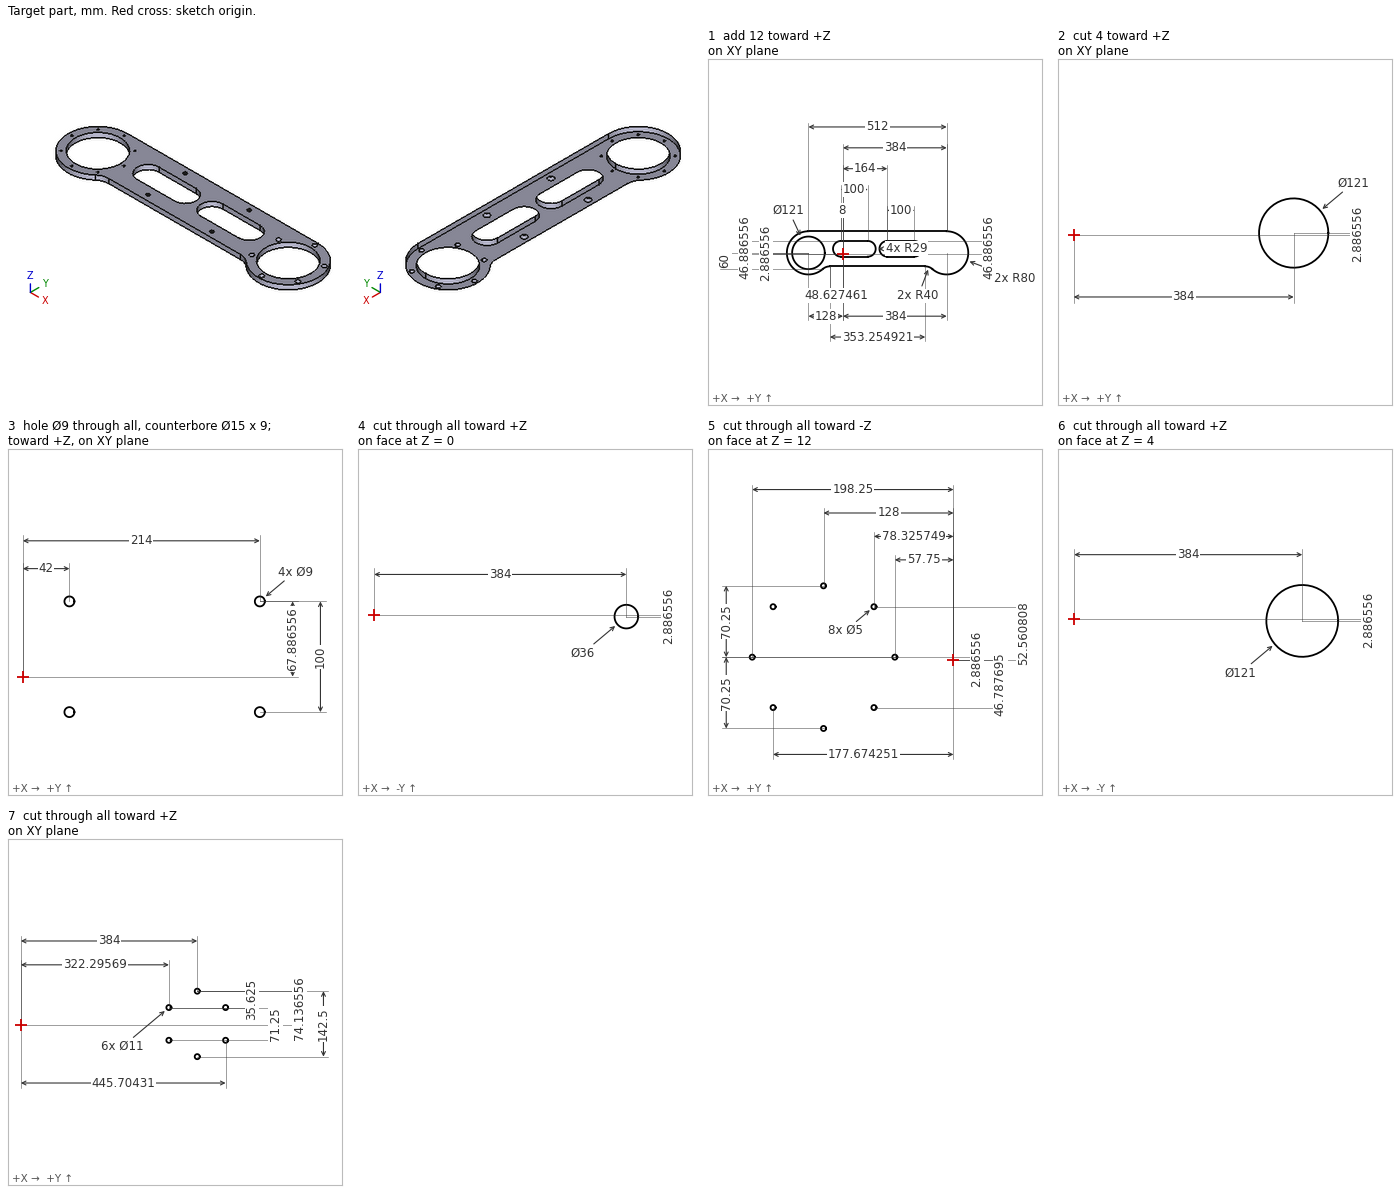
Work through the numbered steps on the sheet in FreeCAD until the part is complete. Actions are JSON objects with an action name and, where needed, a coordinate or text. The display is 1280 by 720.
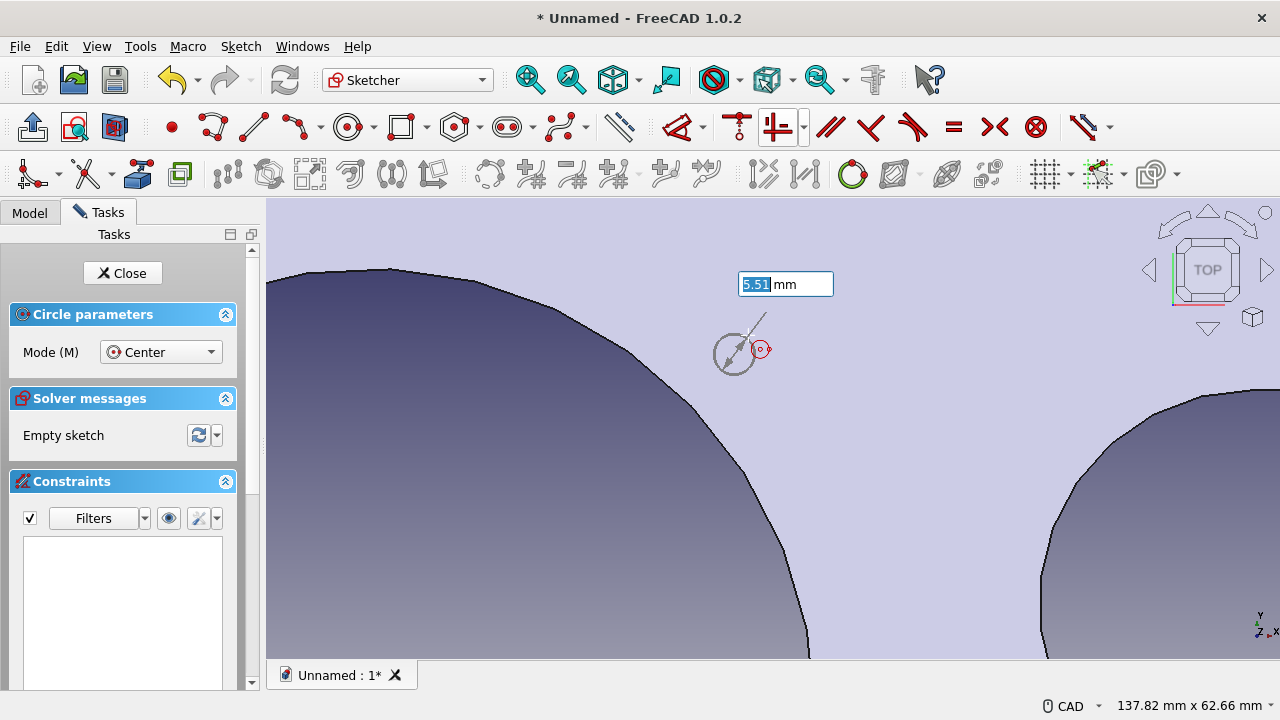
{"action": "left_click", "coordinate": [748, 335]}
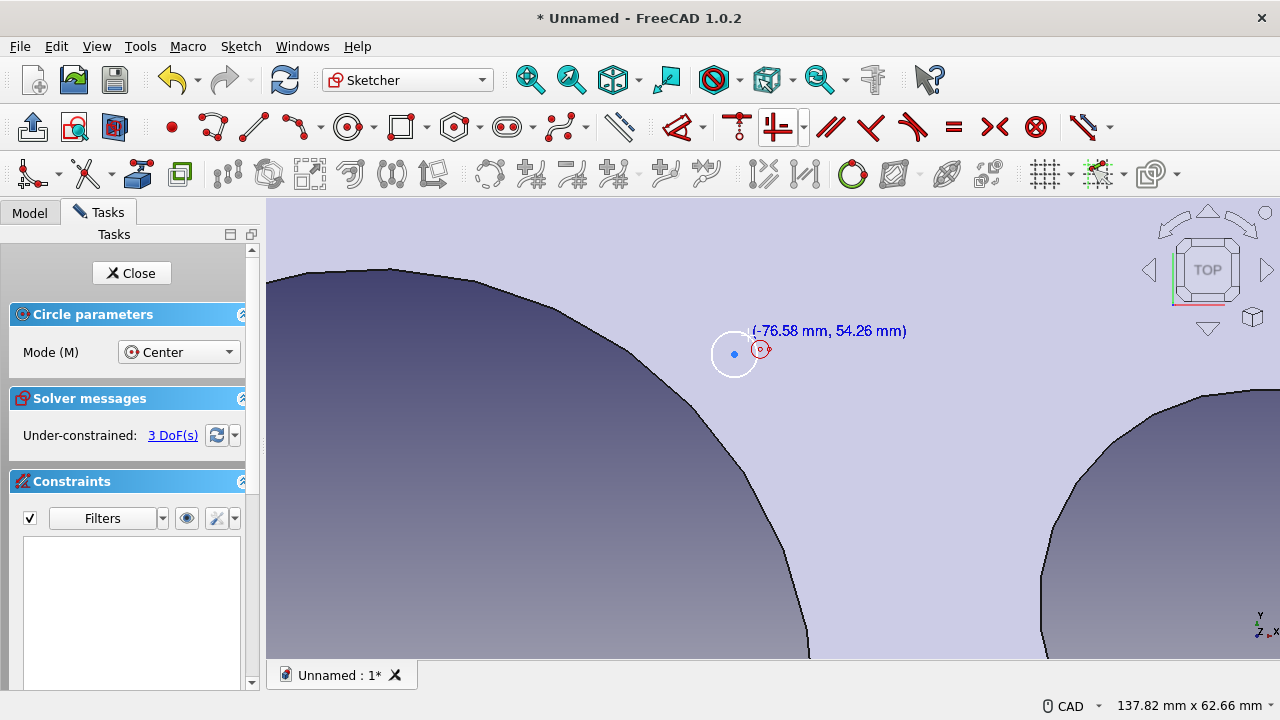
{"action": "scroll", "coordinate": [748, 335], "scroll_direction": "down", "scroll_amount": 7}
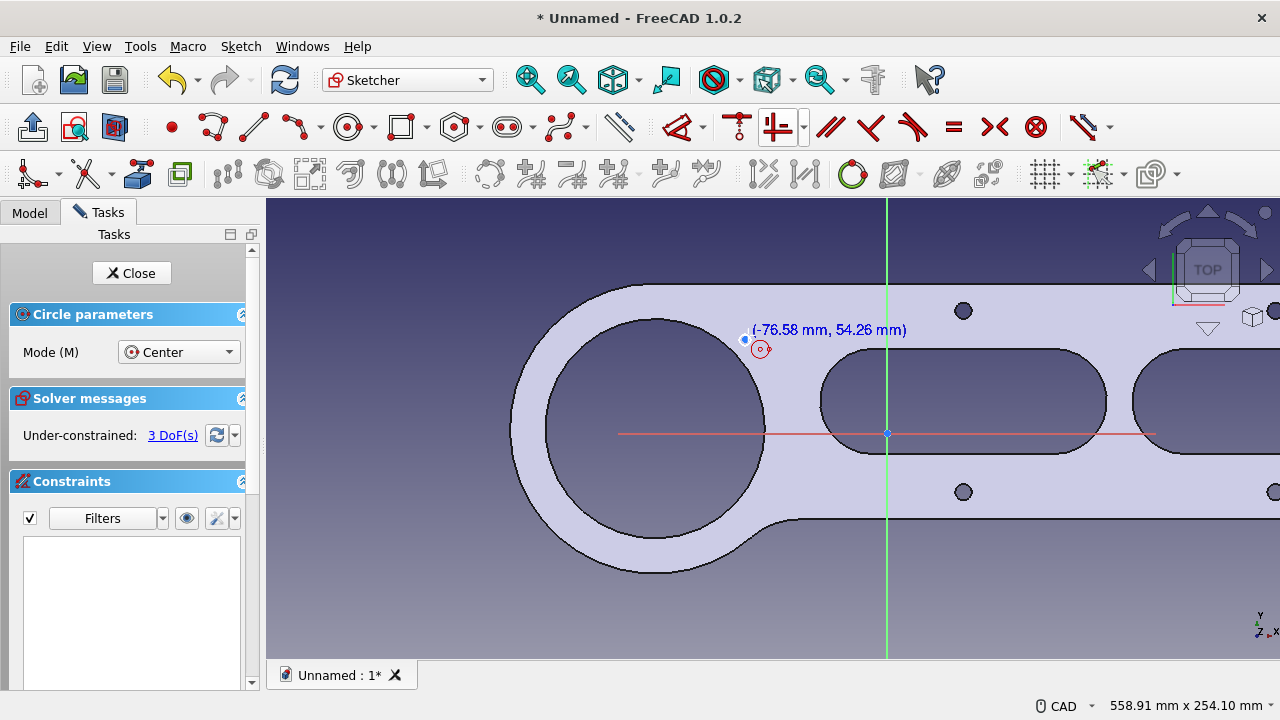
{"action": "scroll", "coordinate": [655, 301], "scroll_direction": "up", "scroll_amount": 9}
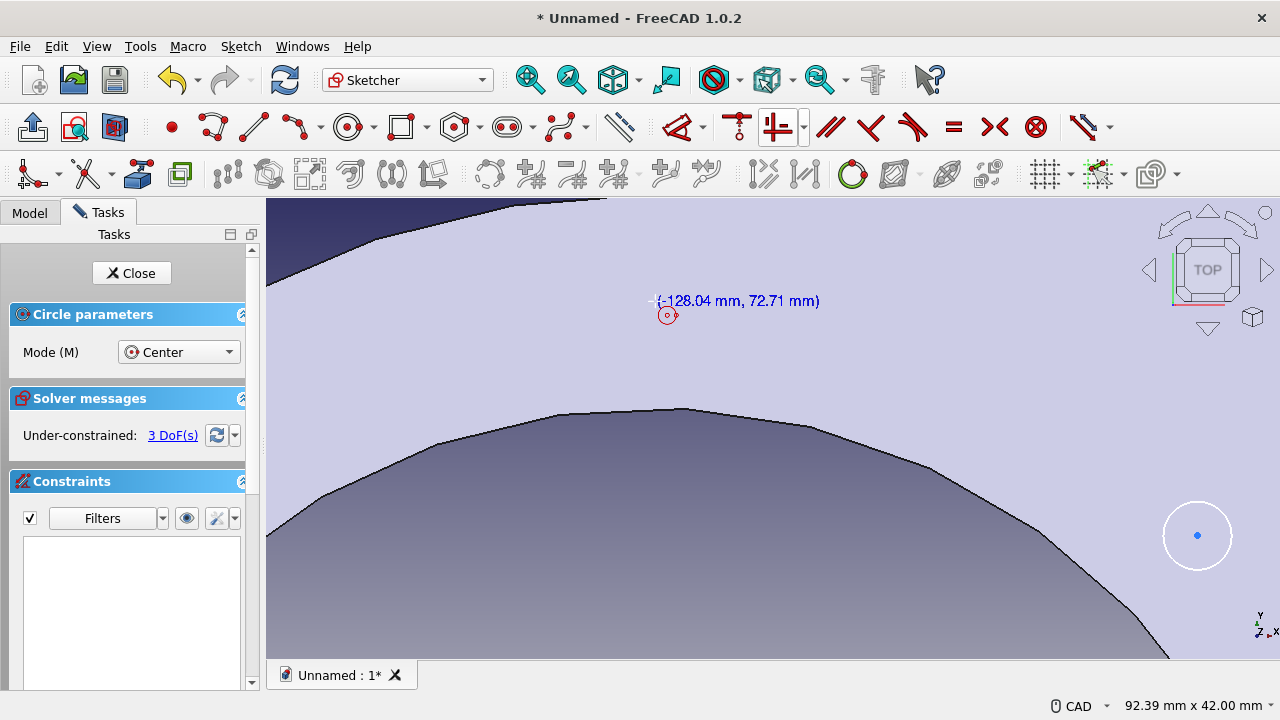
{"action": "scroll", "coordinate": [655, 301], "scroll_direction": "down", "scroll_amount": 9}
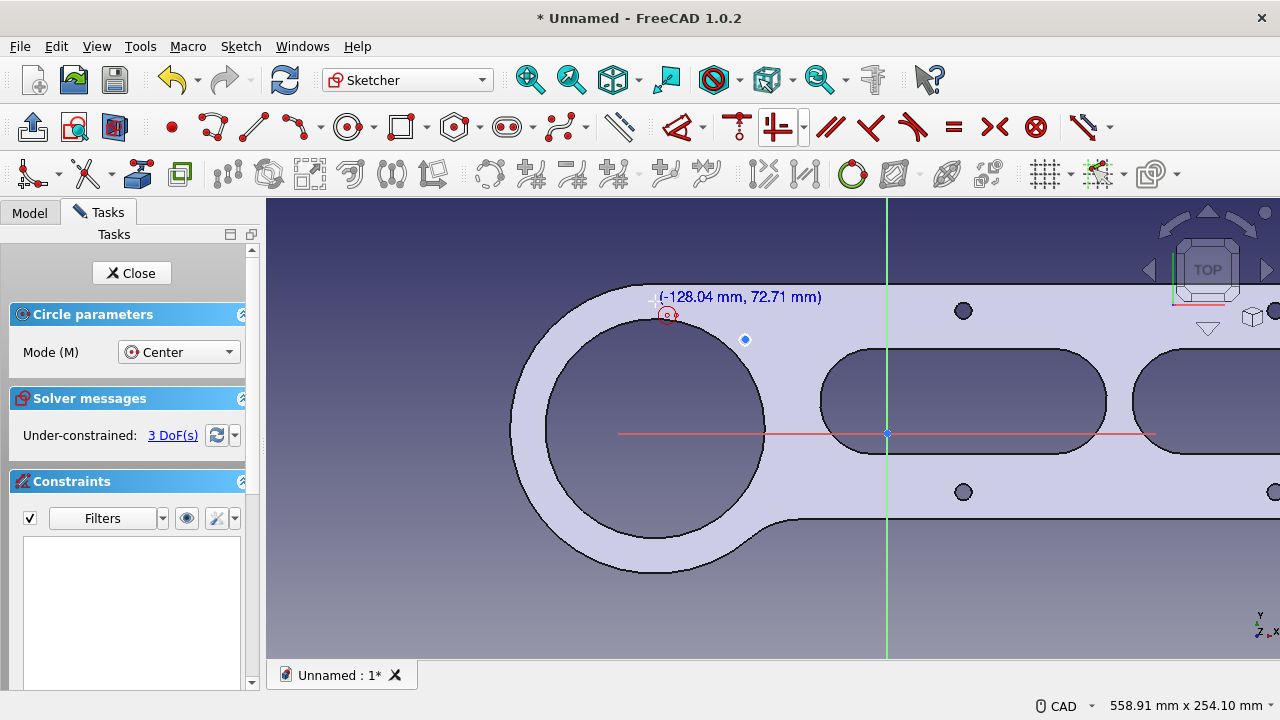
{"action": "left_click", "coordinate": [655, 301]}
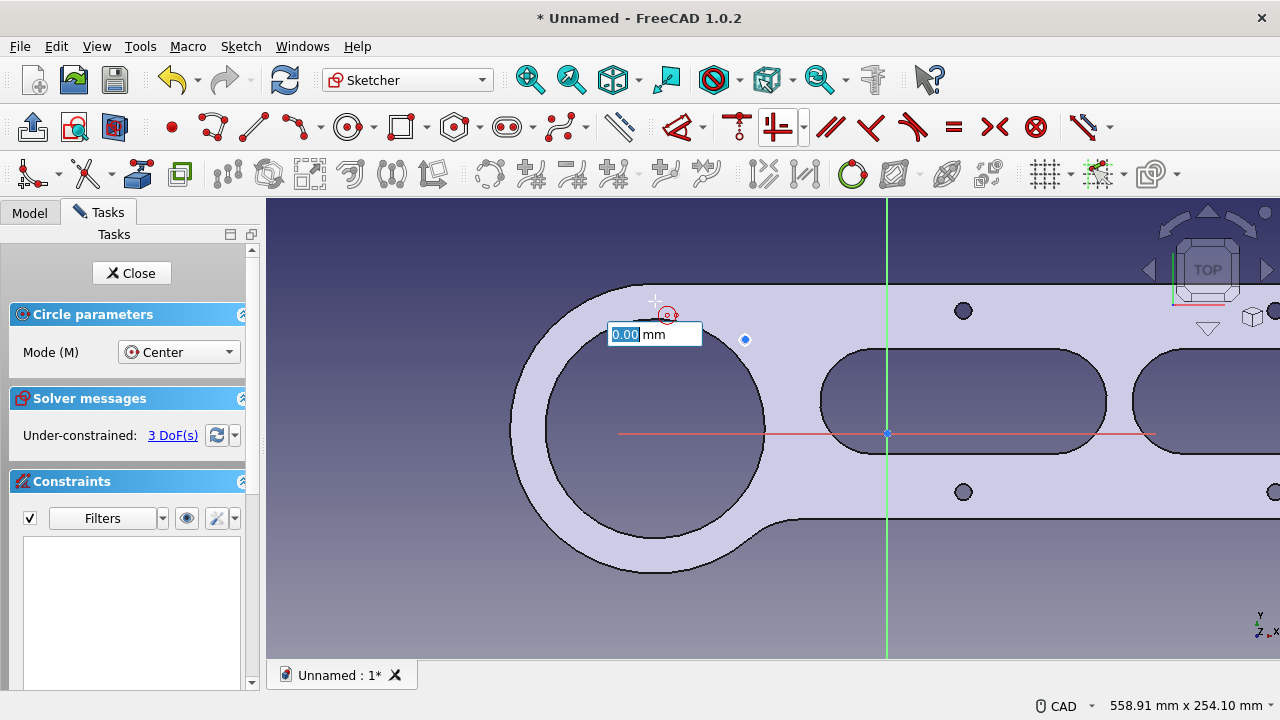
{"action": "scroll", "coordinate": [658, 298], "scroll_direction": "up", "scroll_amount": 7}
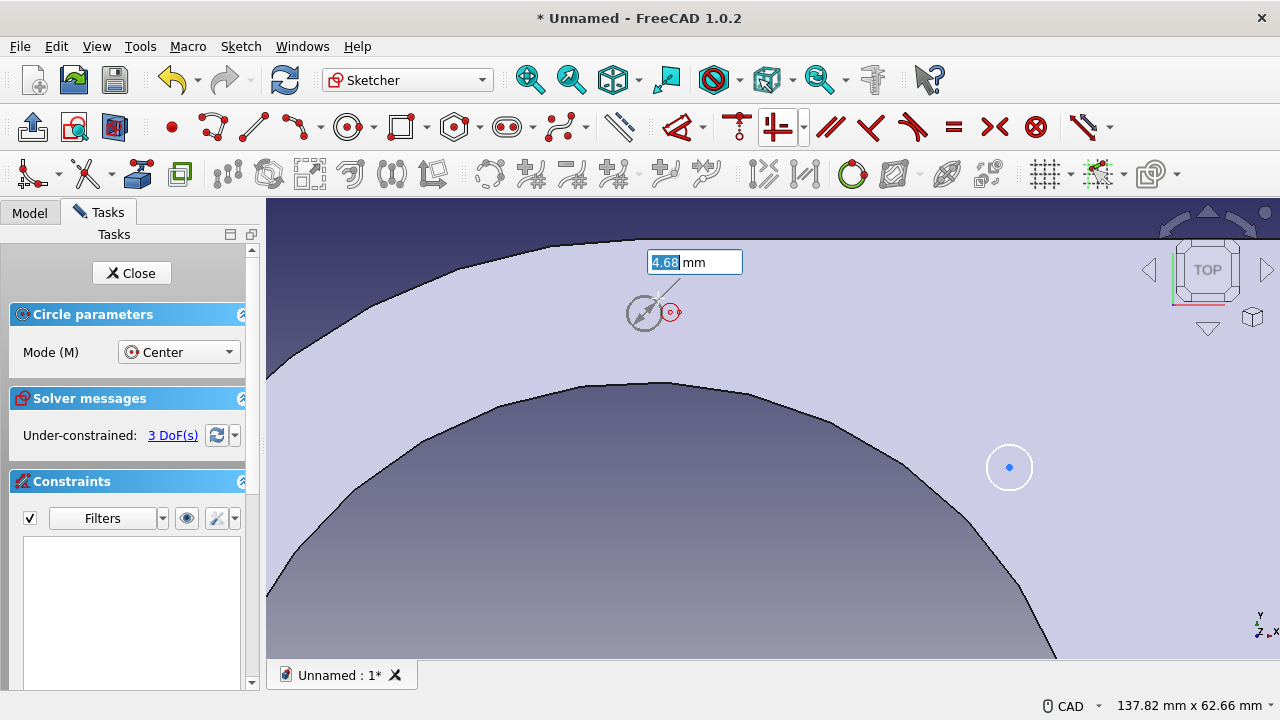
{"action": "left_click", "coordinate": [658, 297]}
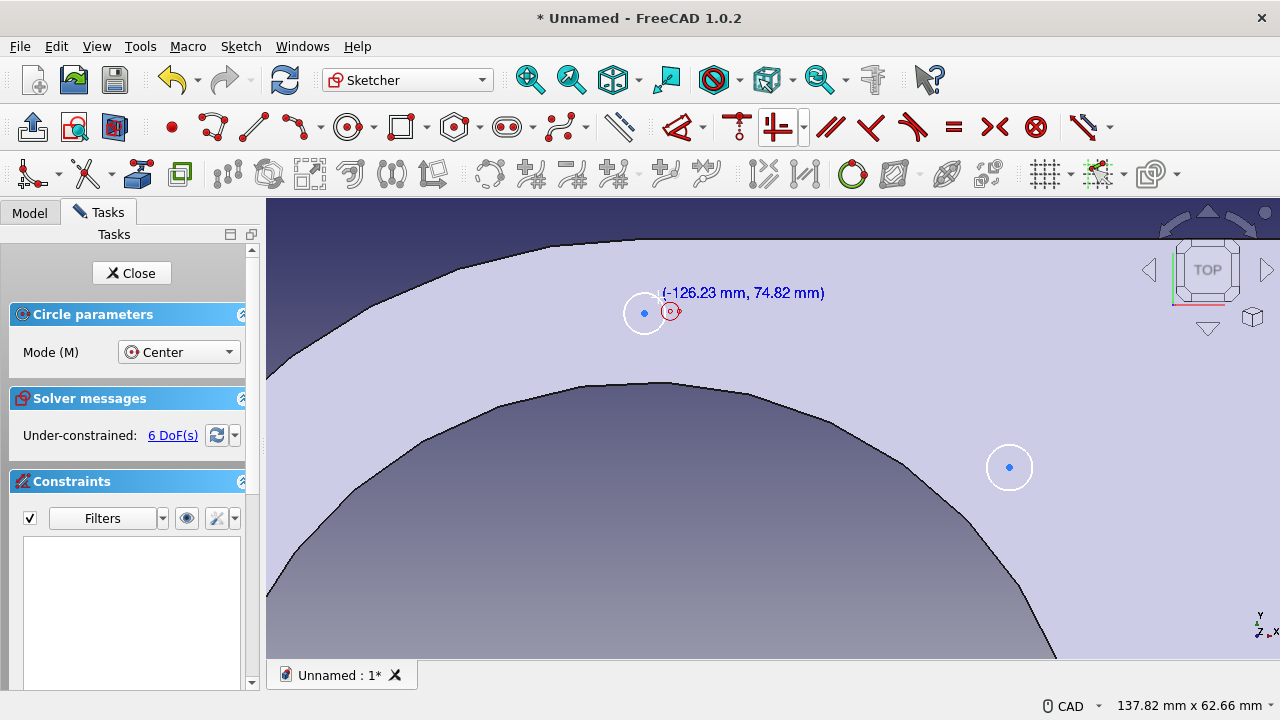
{"action": "scroll", "coordinate": [657, 298], "scroll_direction": "down", "scroll_amount": 7}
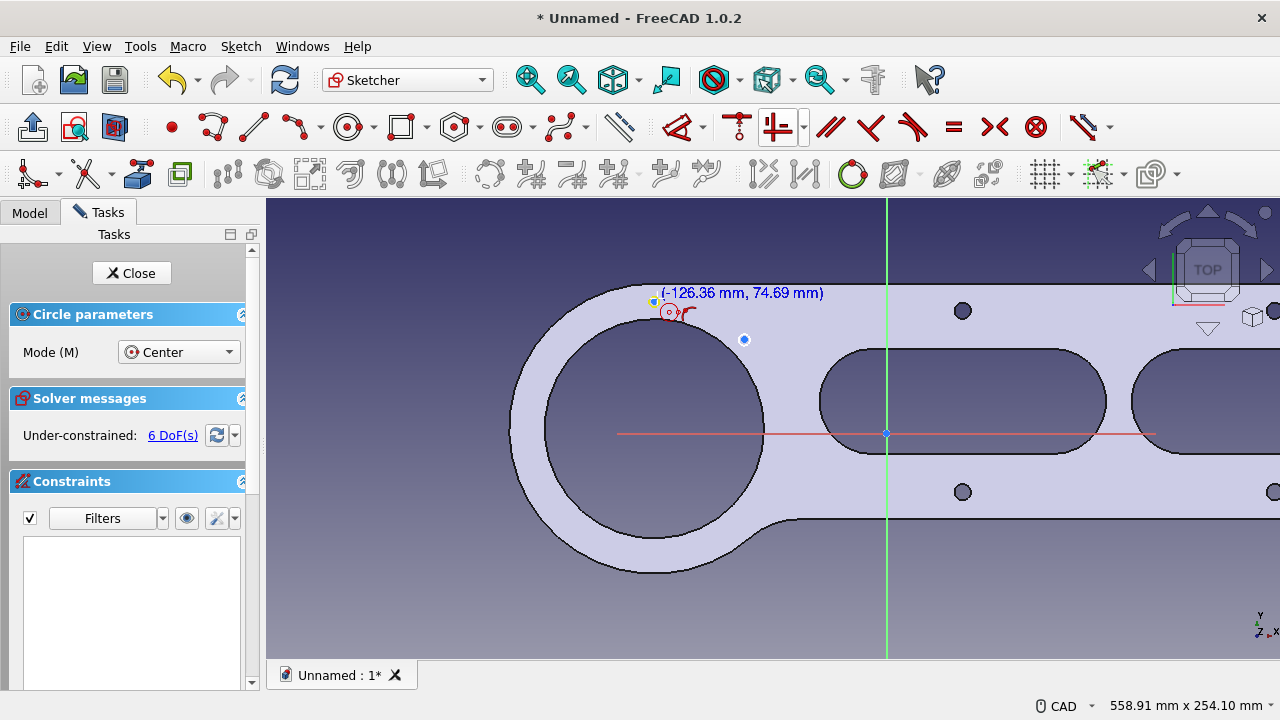
{"action": "scroll", "coordinate": [782, 429], "scroll_direction": "up", "scroll_amount": 9}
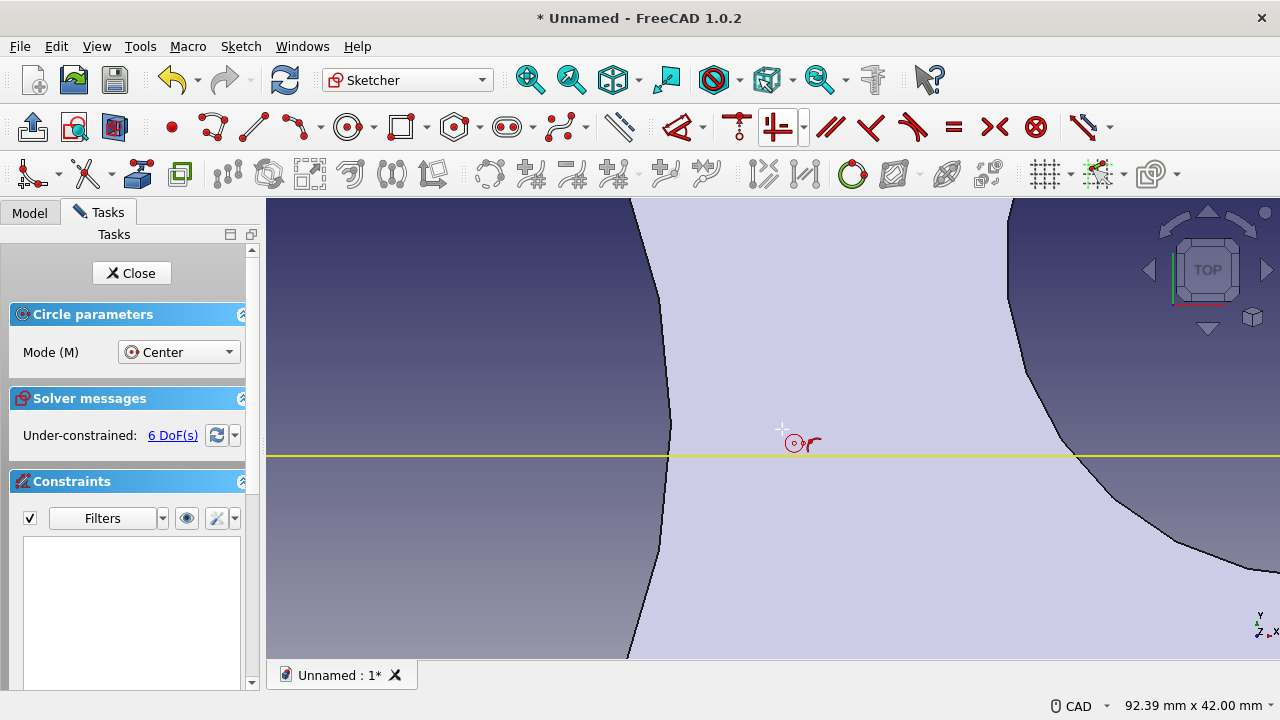
{"action": "left_click", "coordinate": [778, 425]}
{"action": "left_click", "coordinate": [797, 405]}